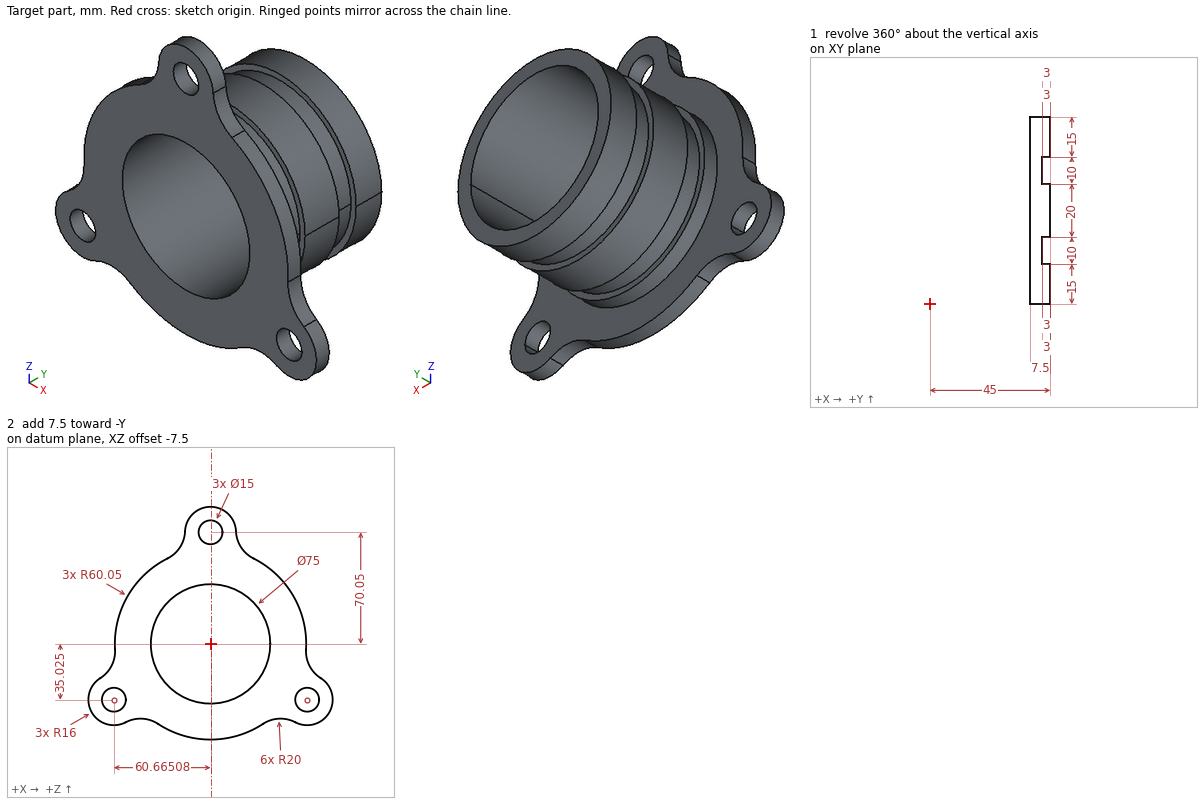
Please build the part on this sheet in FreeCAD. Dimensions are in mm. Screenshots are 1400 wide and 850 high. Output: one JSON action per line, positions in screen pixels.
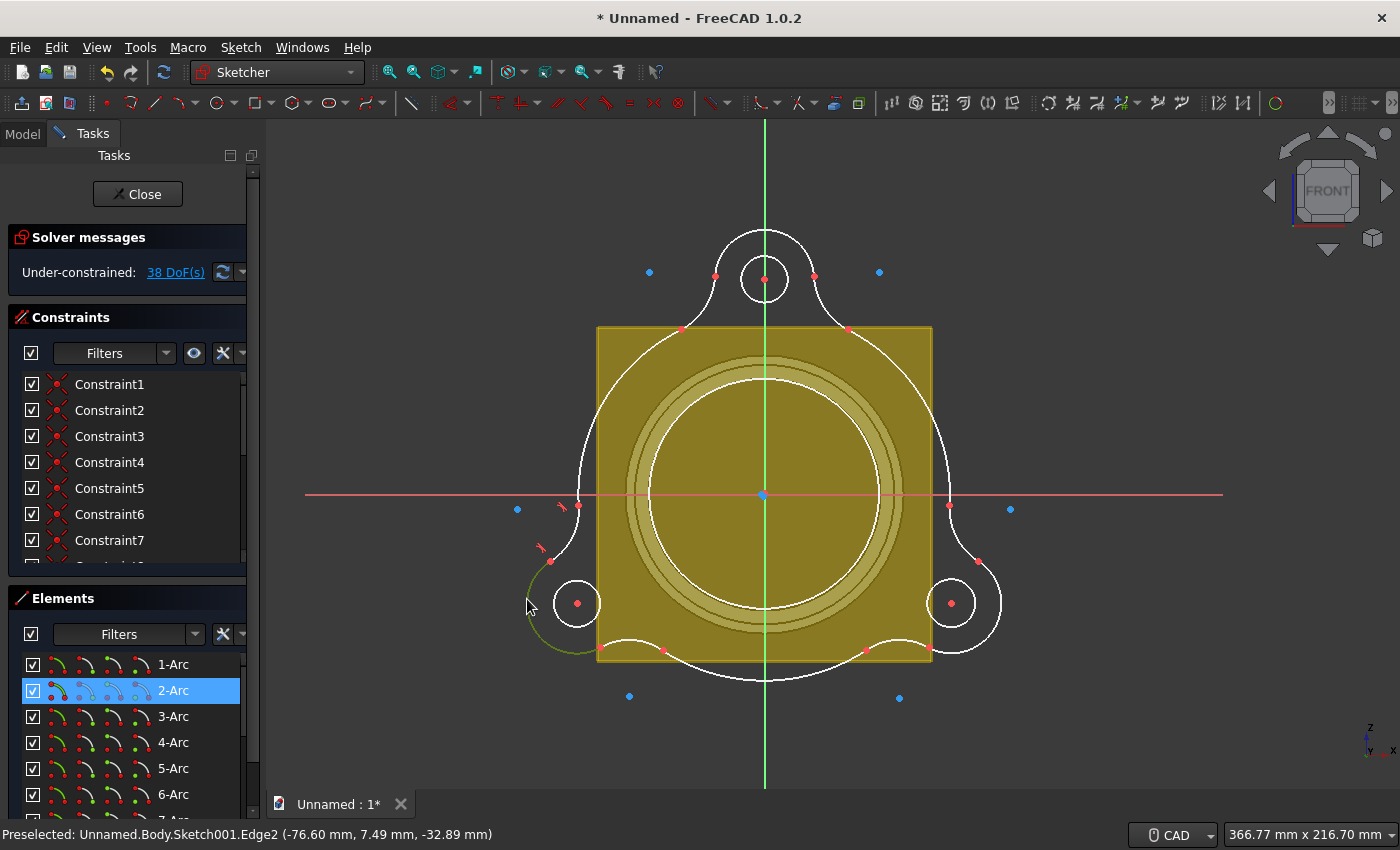
{"action": "left_click", "coordinate": [645, 642]}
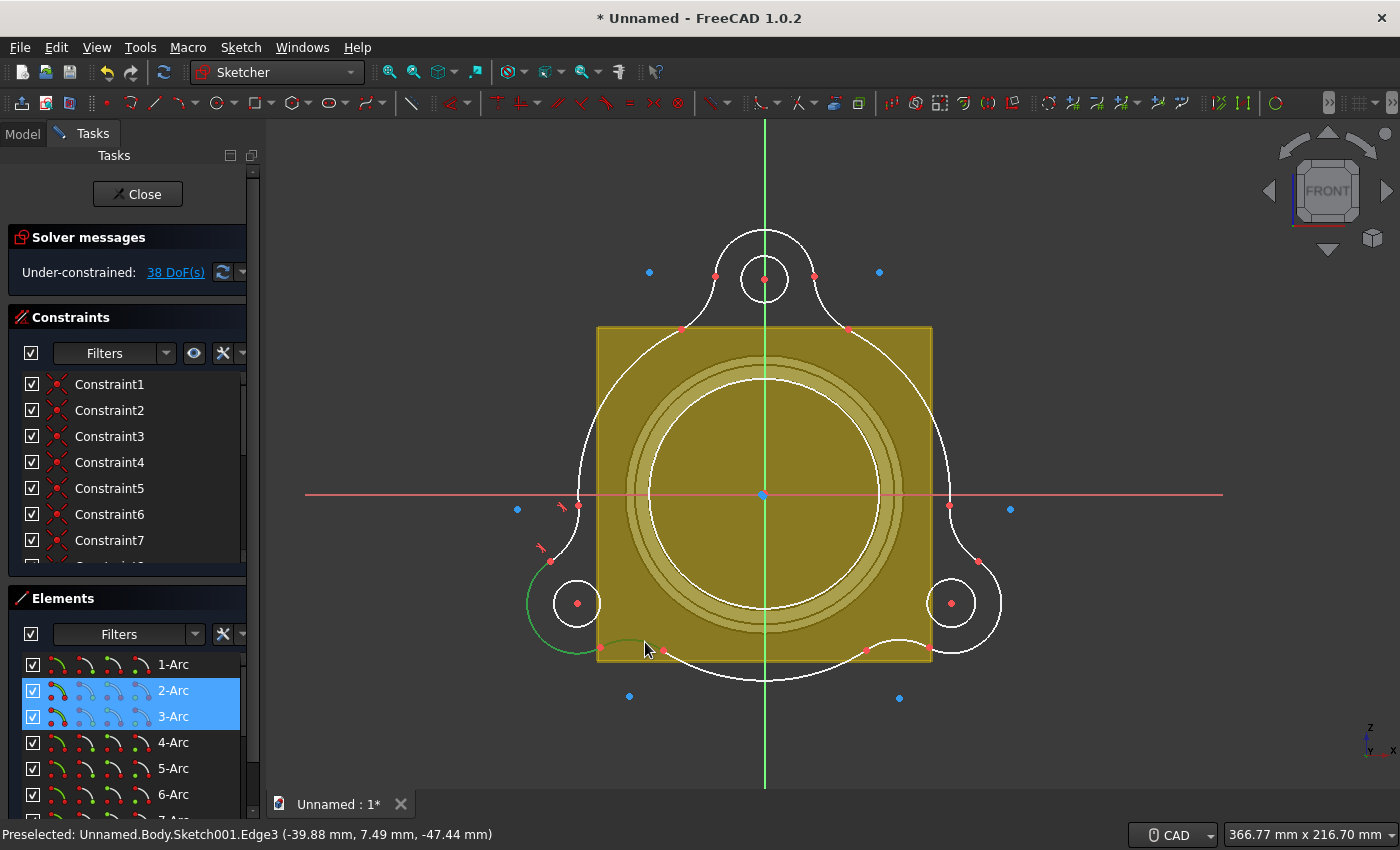
{"action": "left_click", "coordinate": [606, 104]}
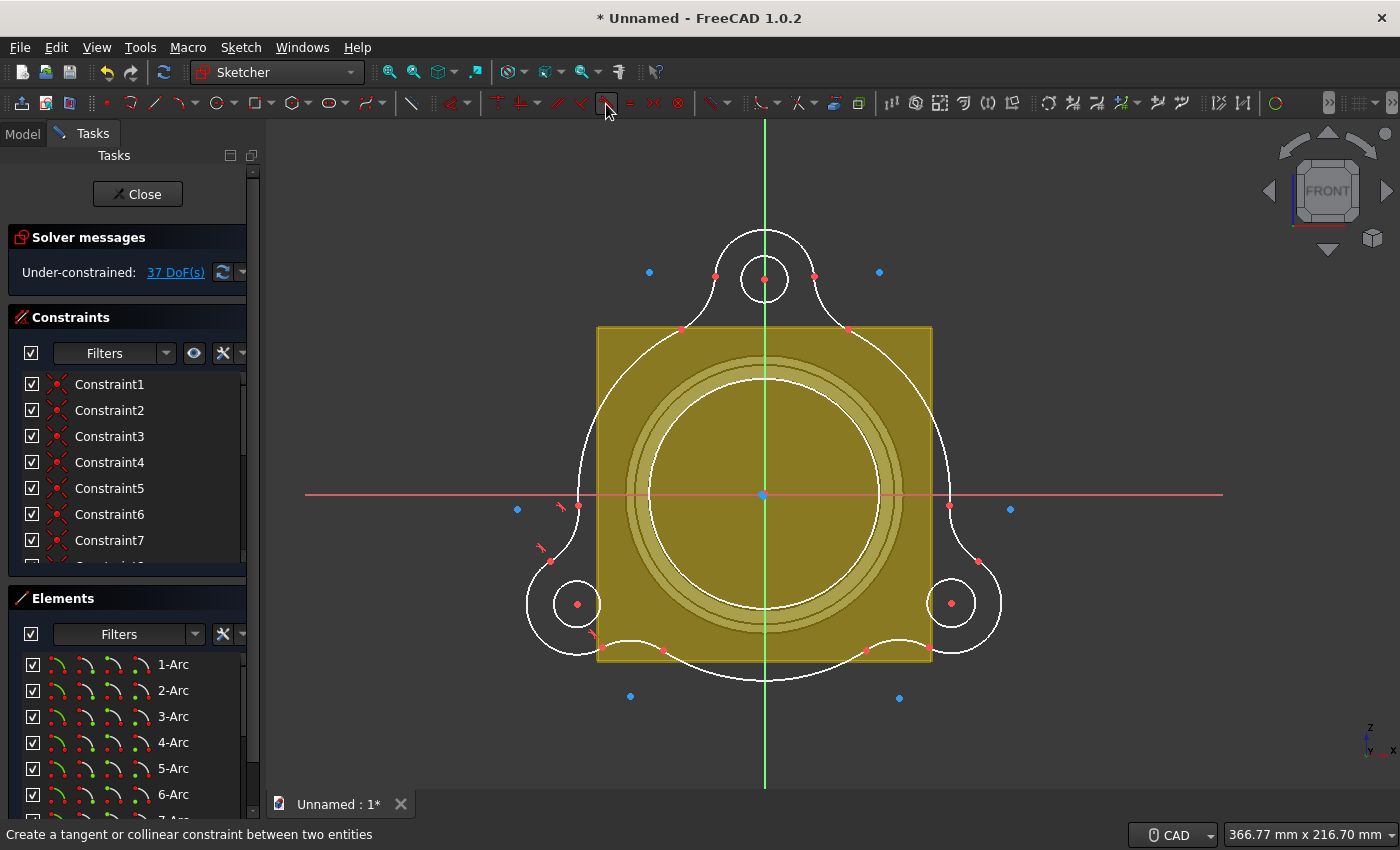
{"action": "left_click", "coordinate": [646, 643]}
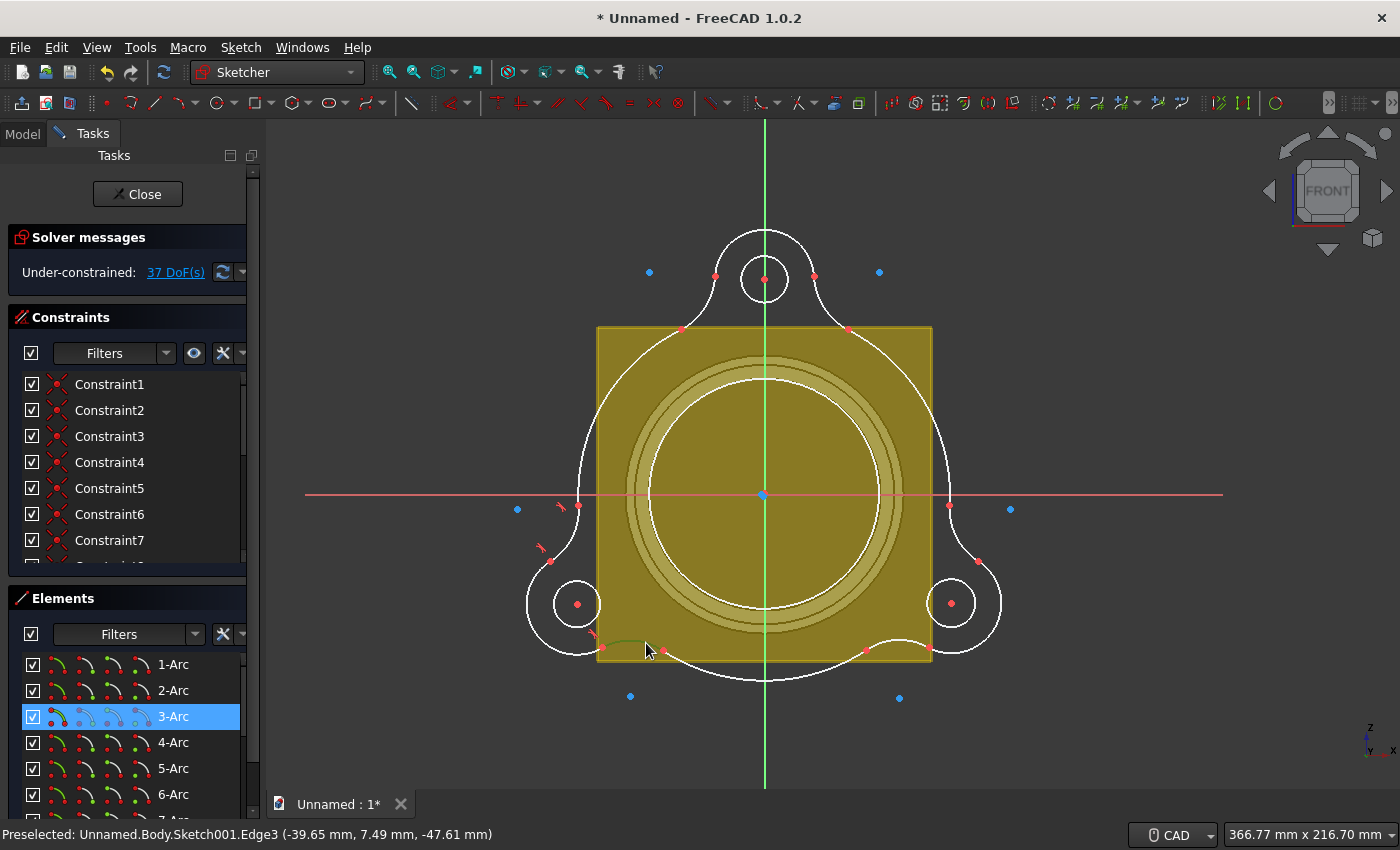
{"action": "left_click", "coordinate": [722, 676]}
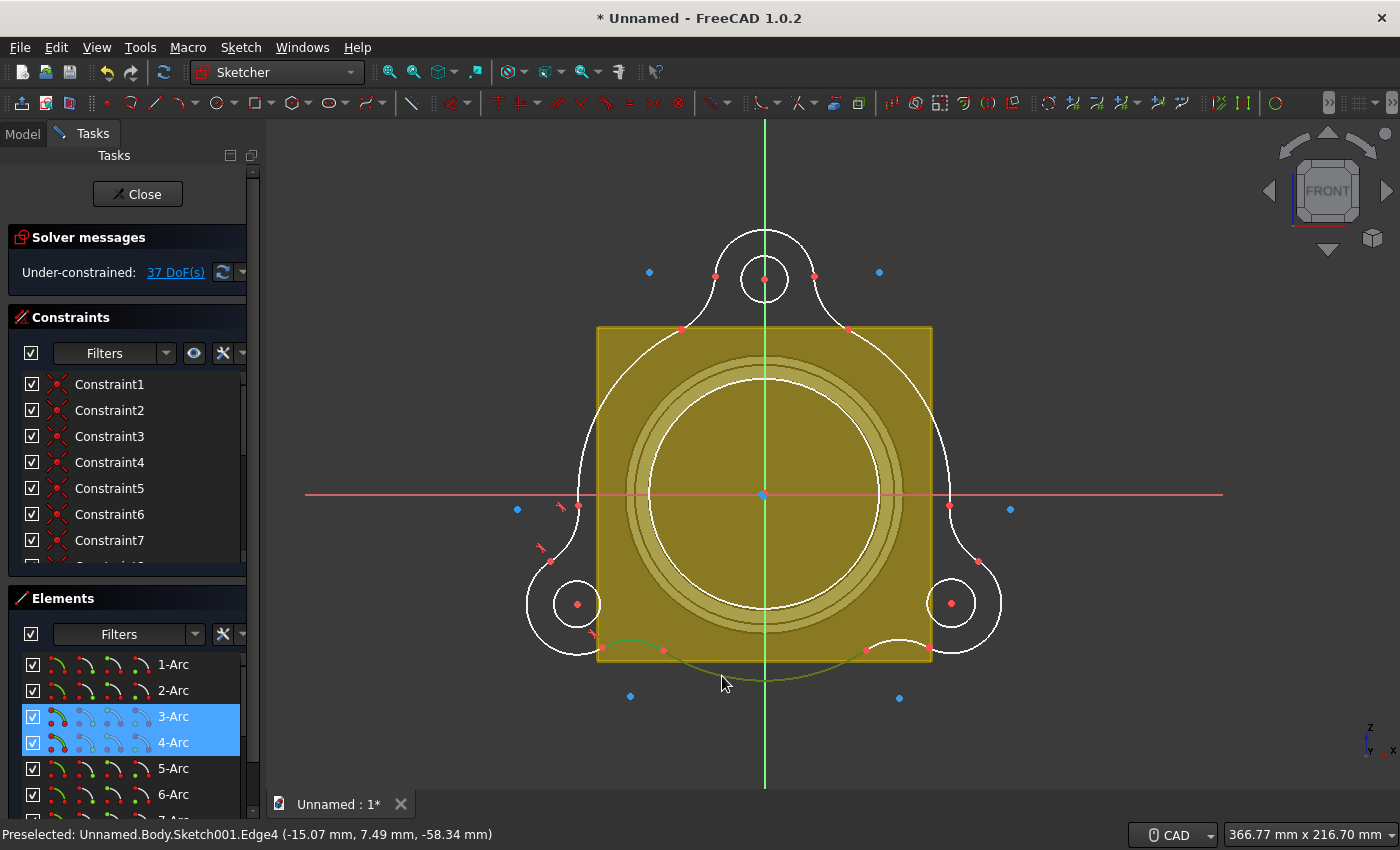
{"action": "left_click", "coordinate": [606, 104]}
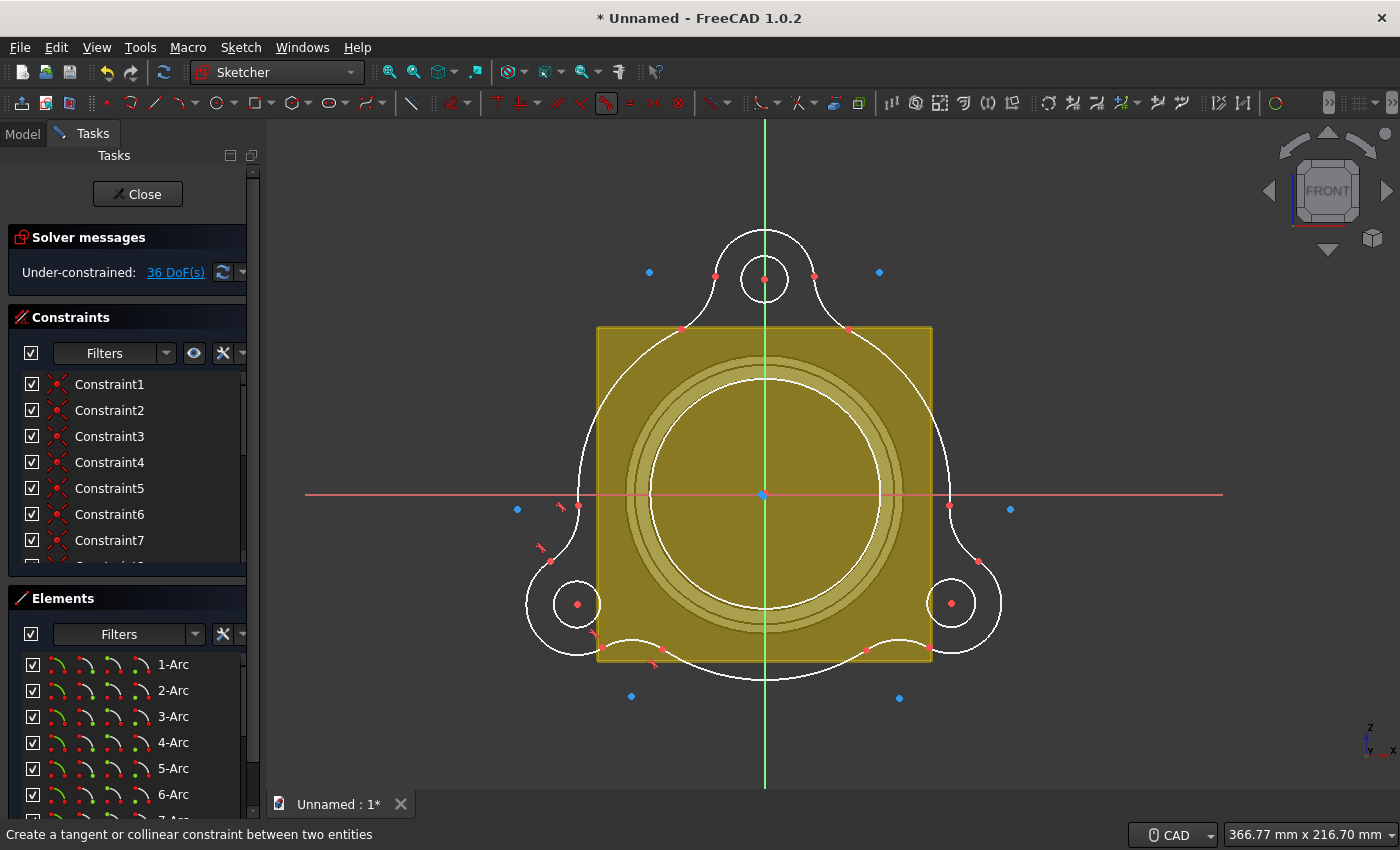
{"action": "left_click", "coordinate": [722, 675]}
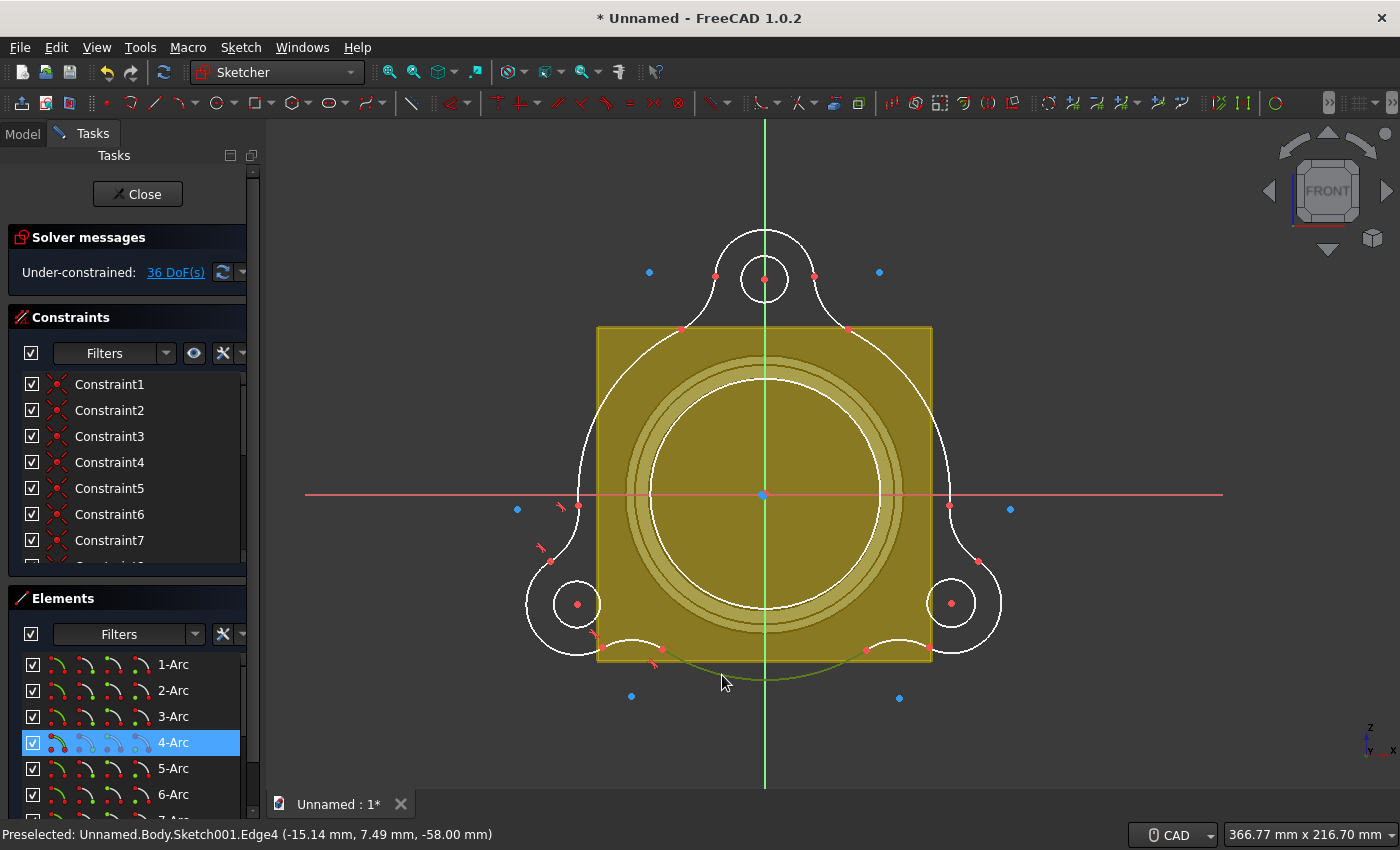
{"action": "left_click", "coordinate": [910, 641]}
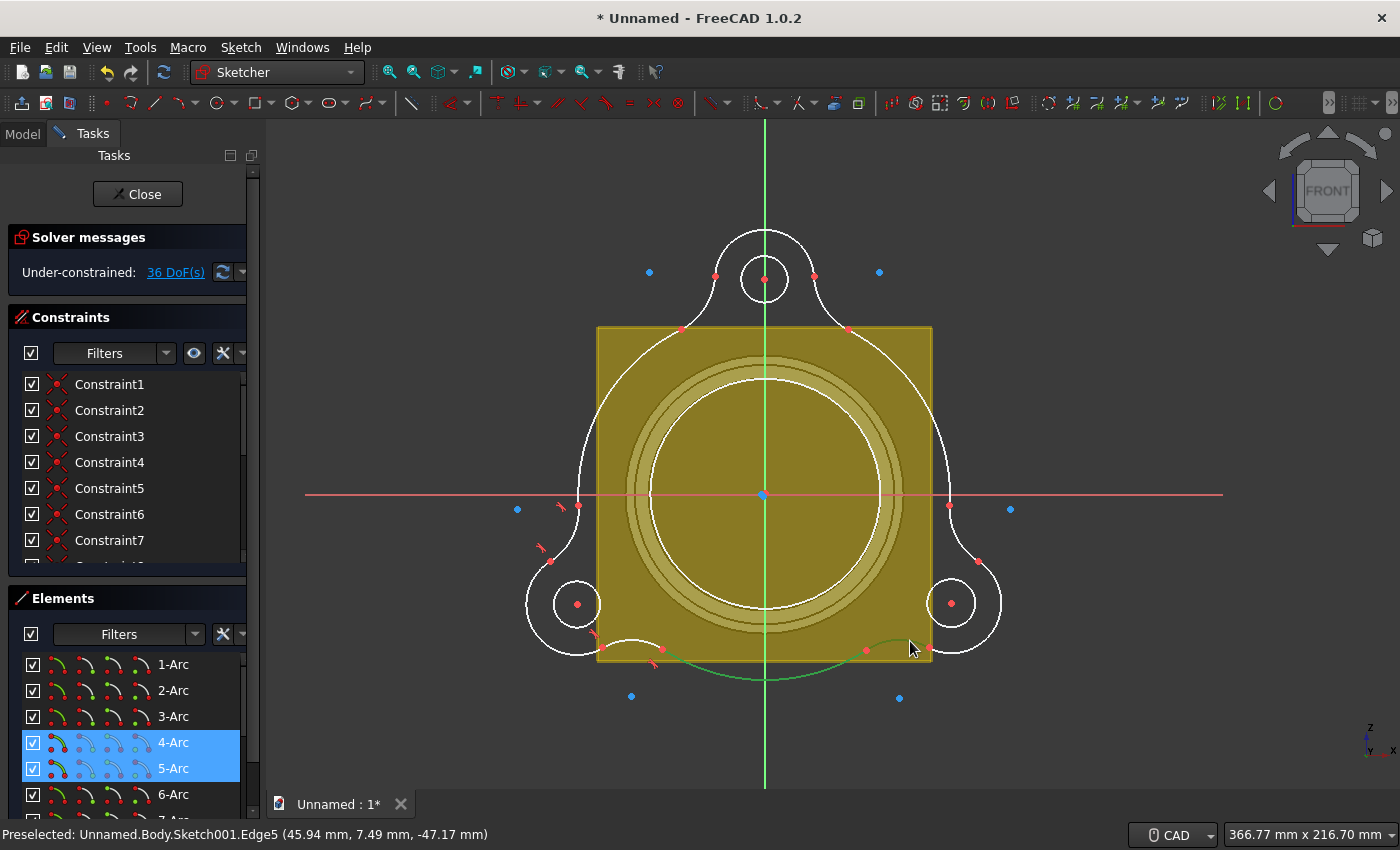
{"action": "left_click", "coordinate": [606, 104]}